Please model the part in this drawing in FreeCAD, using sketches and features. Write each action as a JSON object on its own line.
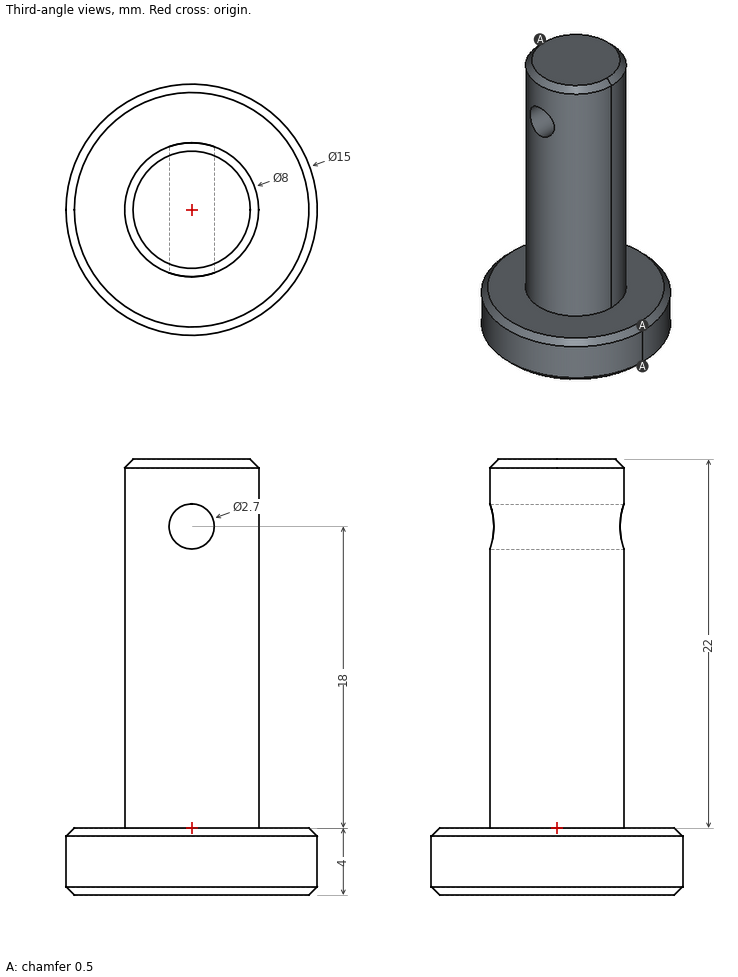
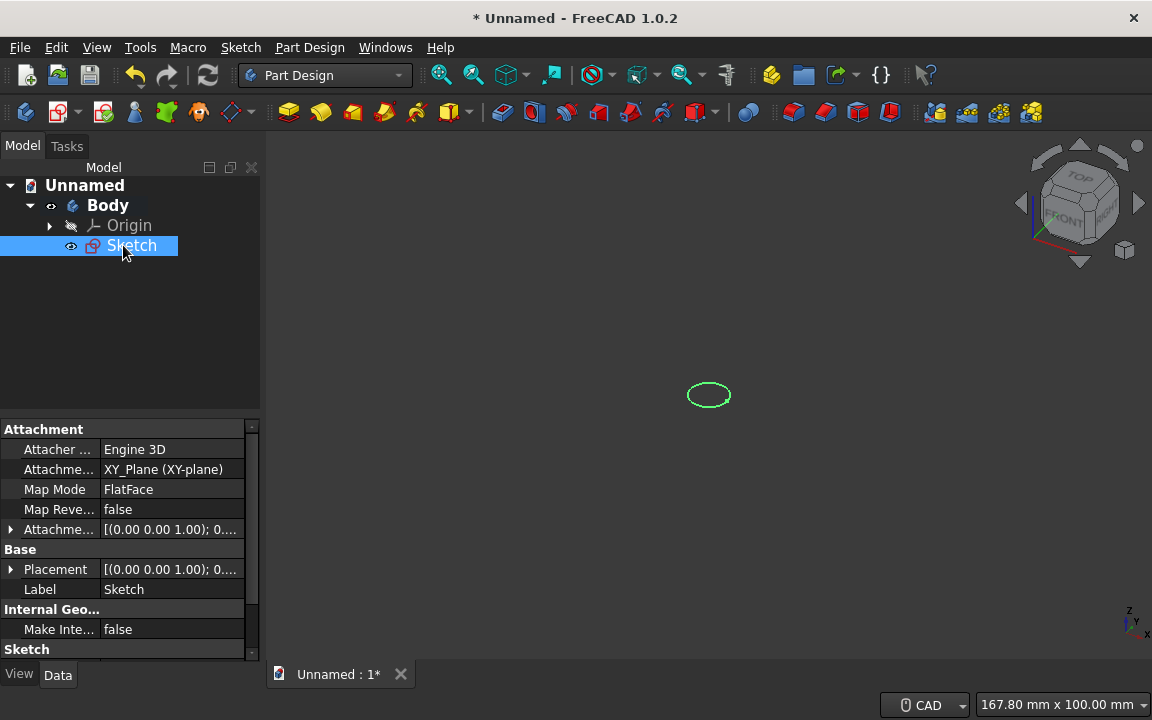
{"action": "left_click", "coordinate": [290, 112]}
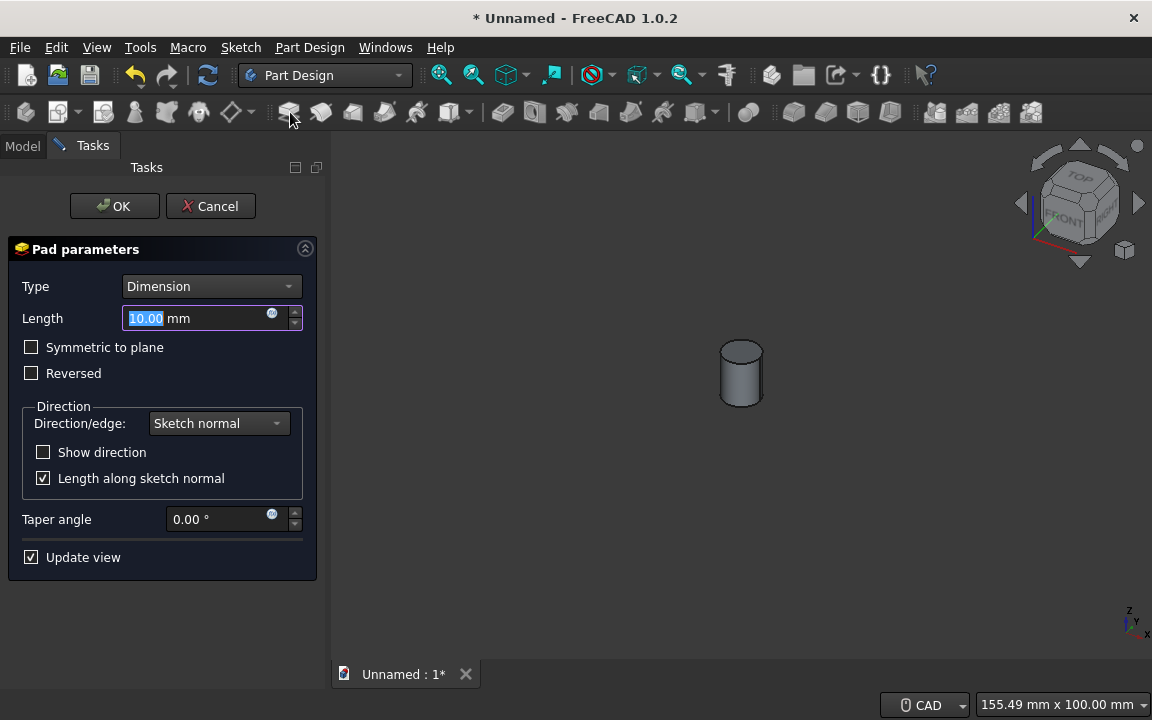
{"action": "type", "text": "22"}
{"action": "key", "text": "Tab"}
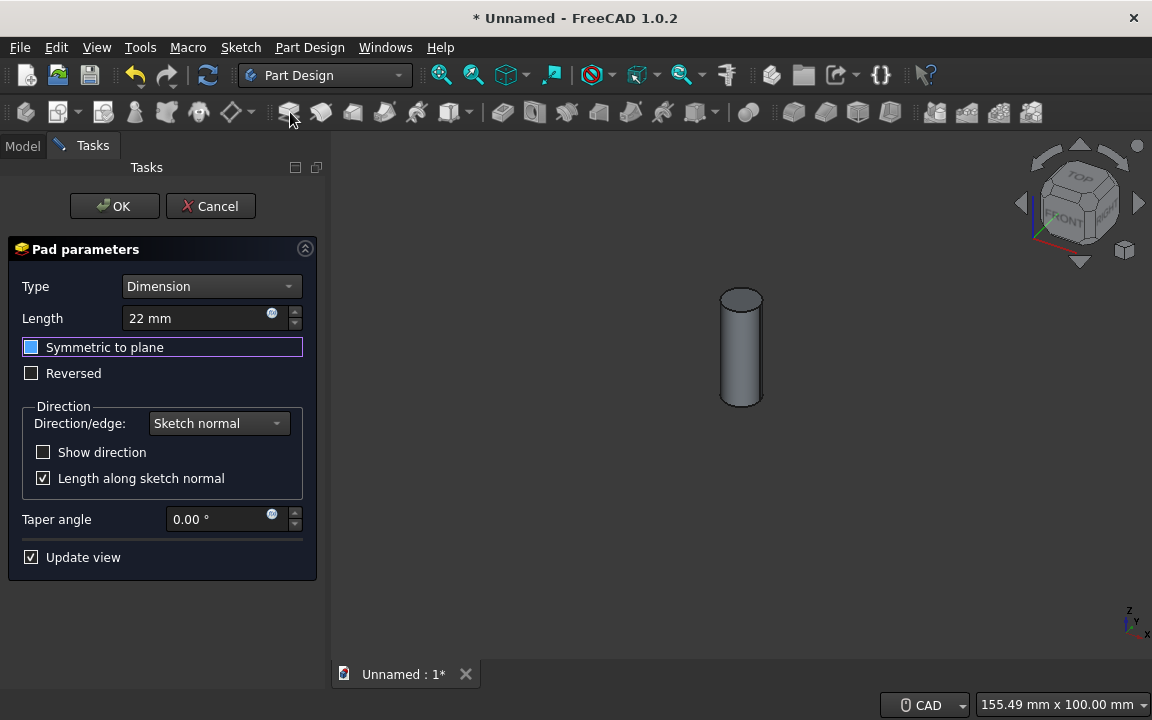
{"action": "left_click", "coordinate": [115, 206]}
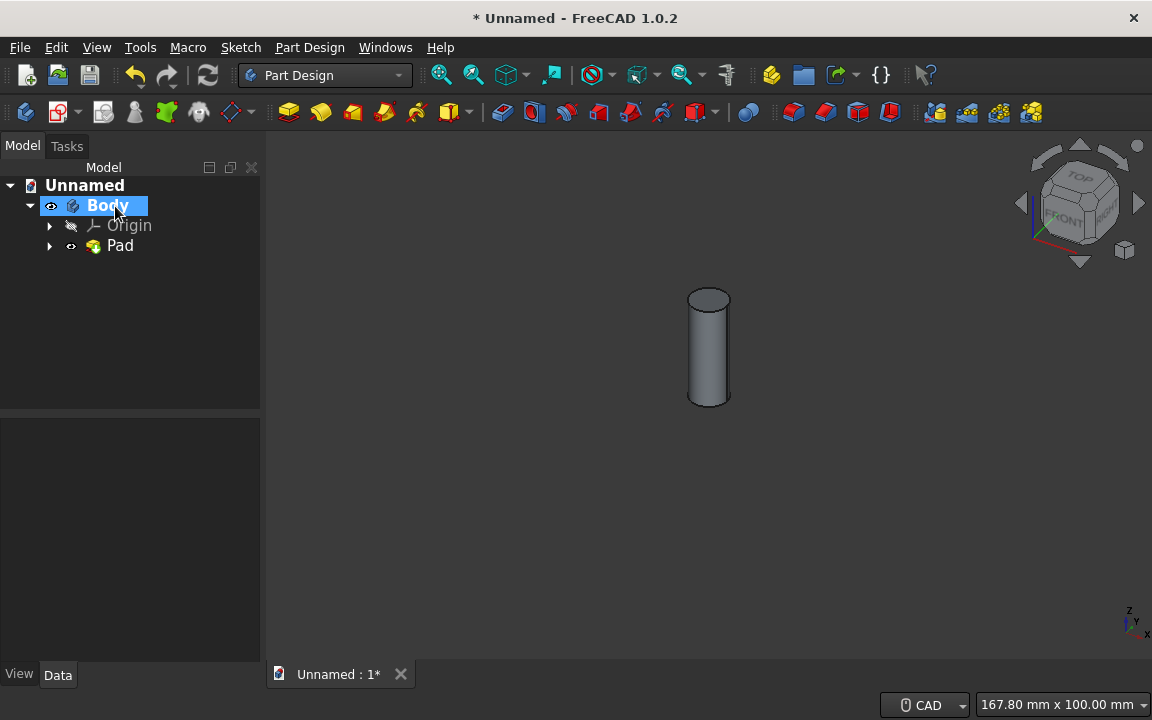
{"action": "left_click", "coordinate": [442, 76]}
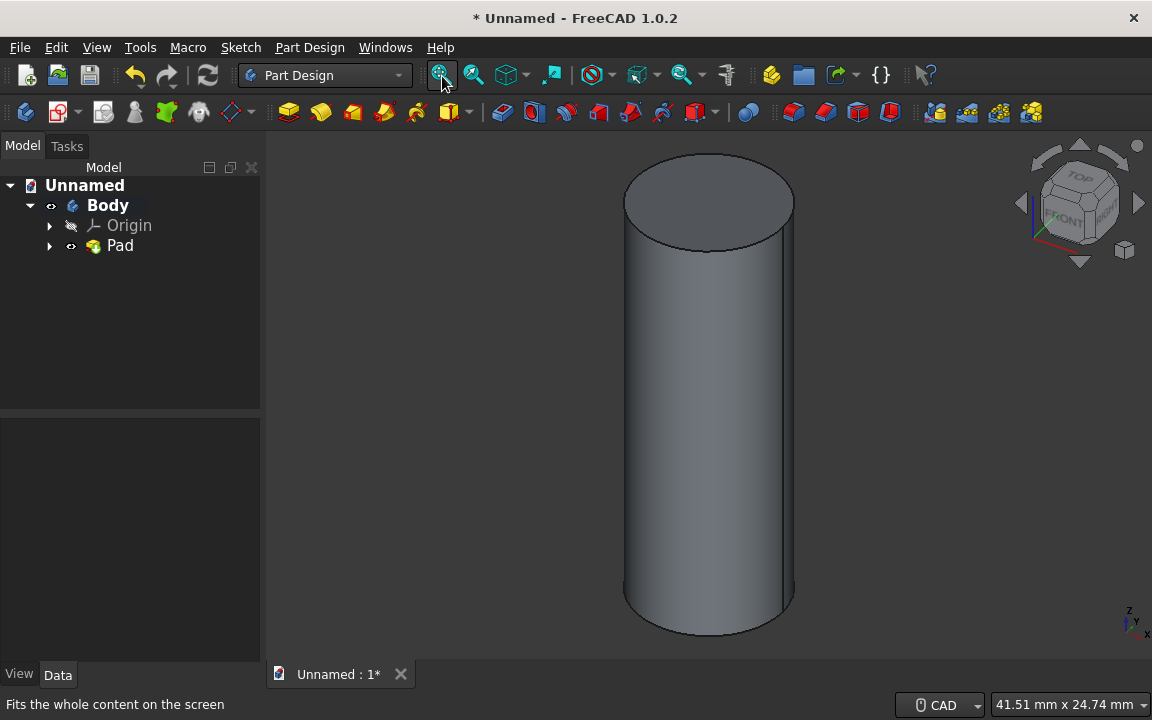
{"action": "key", "text": "5"}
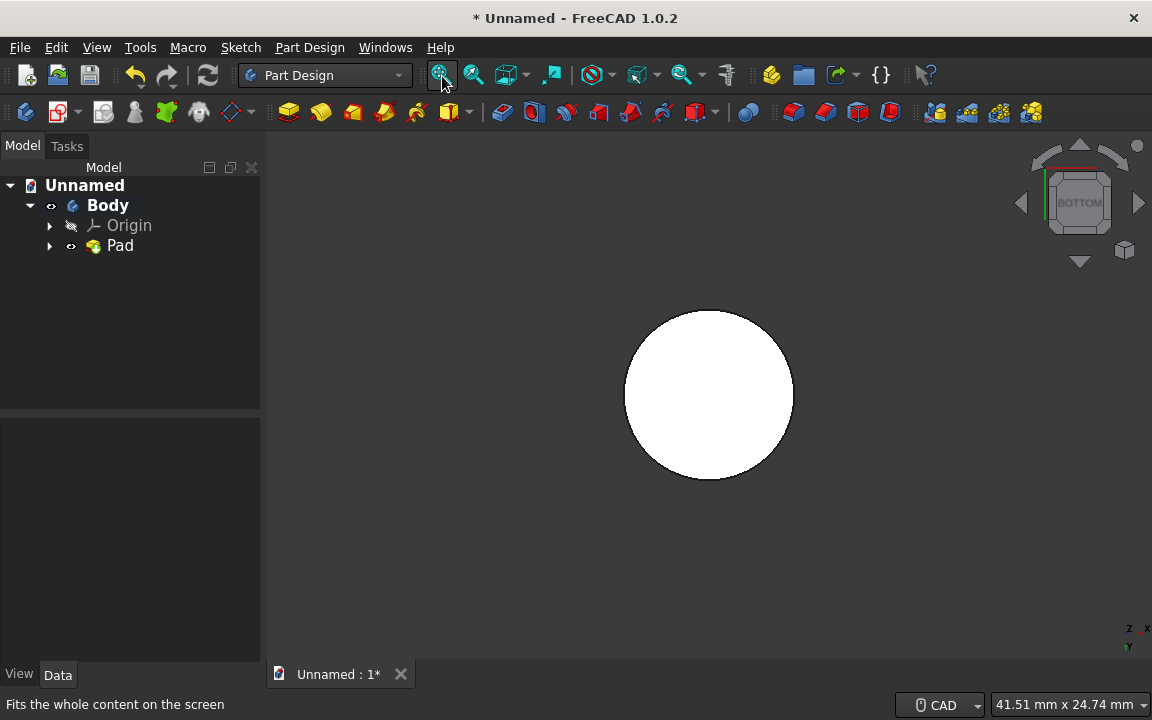
{"action": "left_click", "coordinate": [442, 76]}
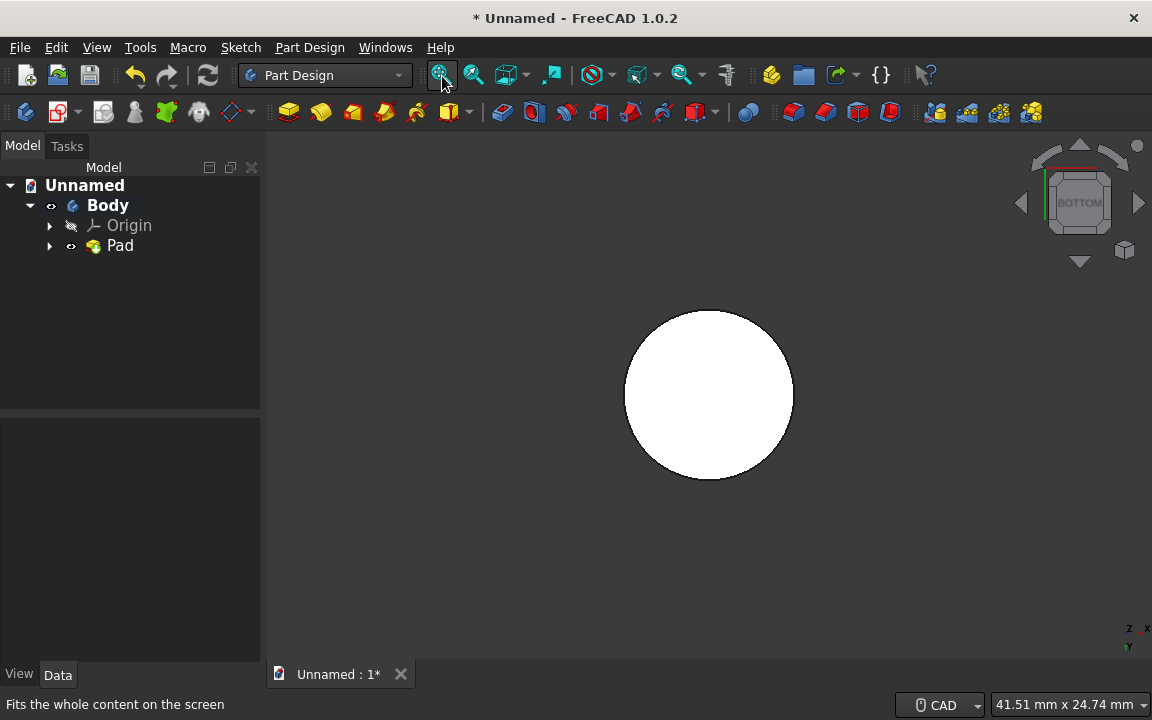
{"action": "left_click", "coordinate": [709, 394]}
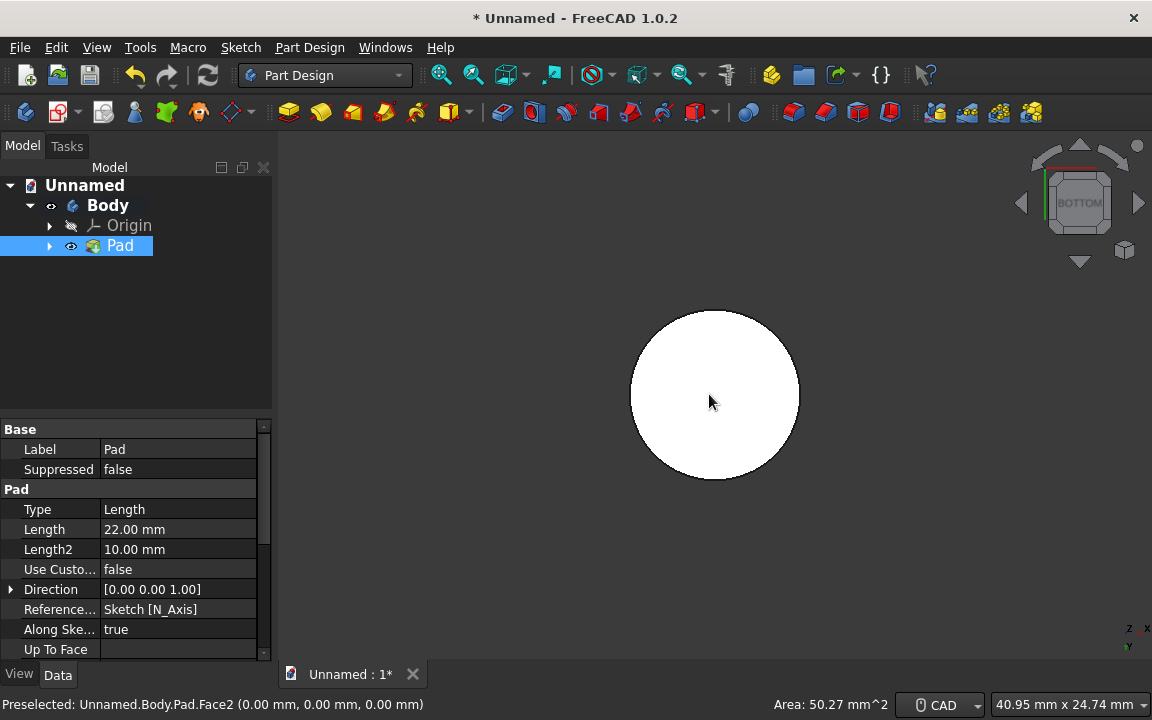
{"action": "left_click", "coordinate": [58, 112]}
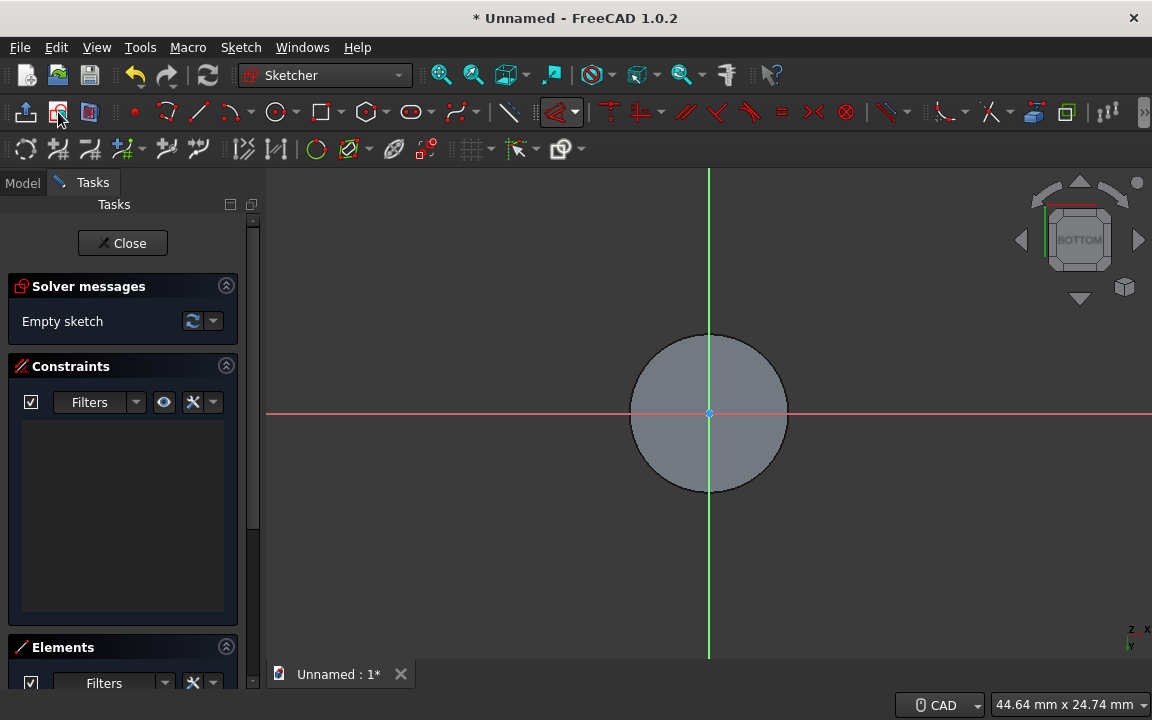
{"action": "key", "text": "g c"}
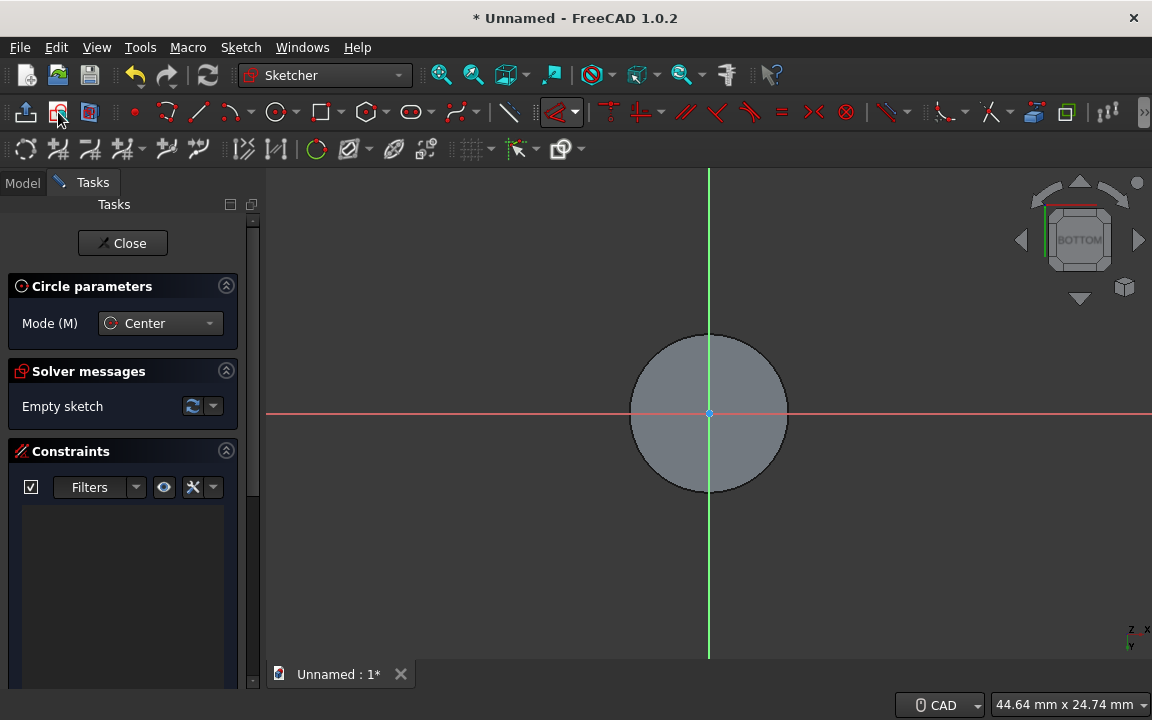
{"action": "left_click", "coordinate": [709, 414]}
{"action": "left_click", "coordinate": [814, 308]}
{"action": "key", "text": "Escape"}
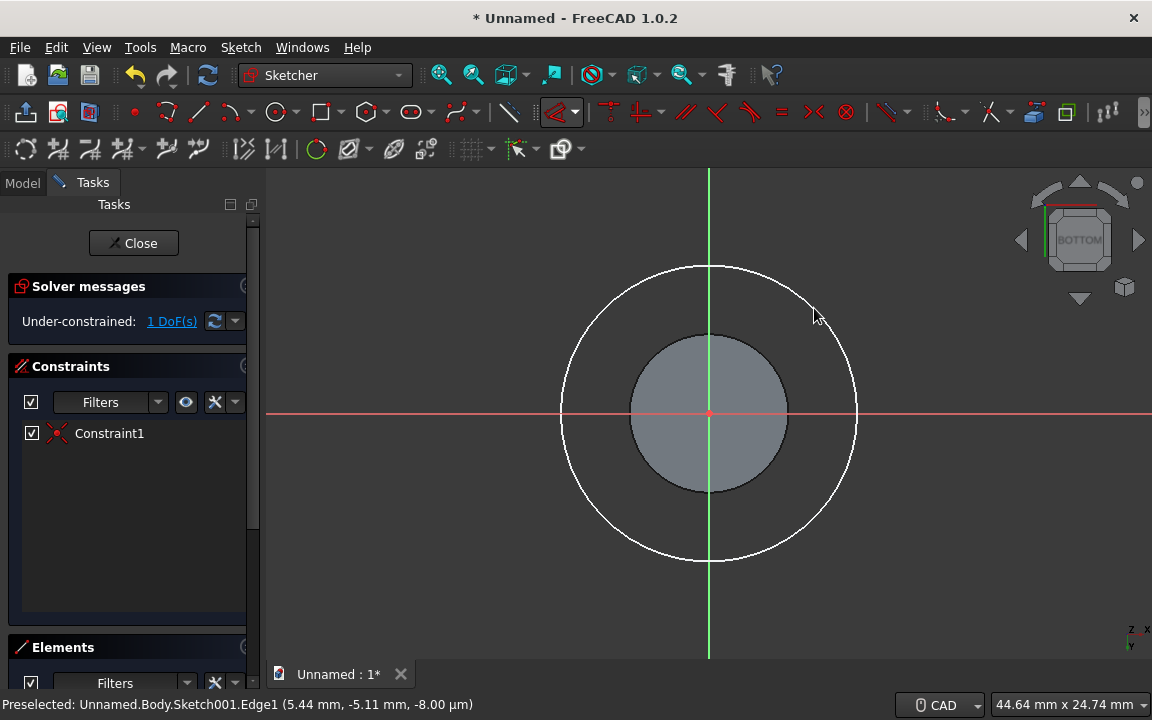
{"action": "left_click", "coordinate": [813, 308]}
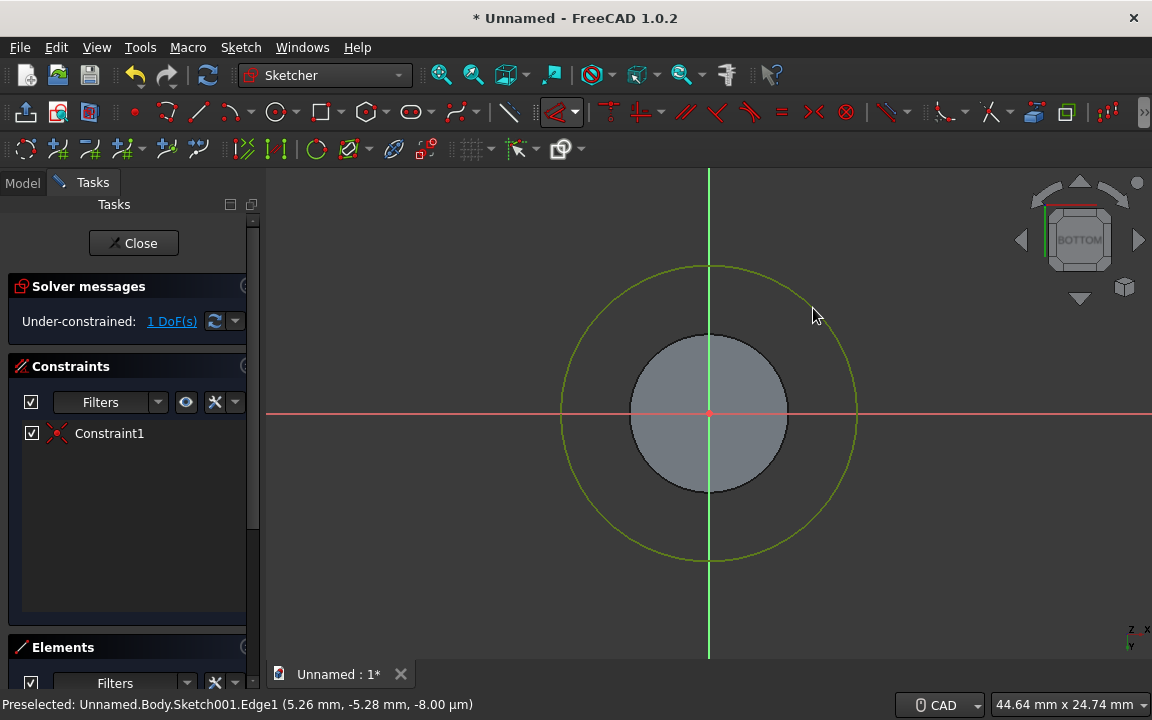
{"action": "left_click", "coordinate": [578, 112]}